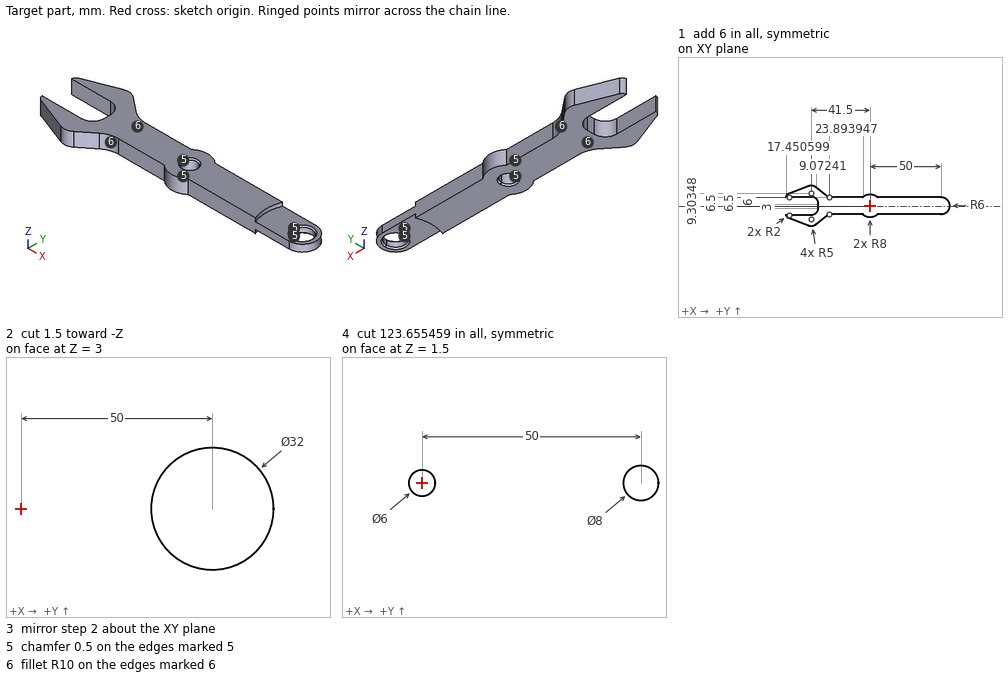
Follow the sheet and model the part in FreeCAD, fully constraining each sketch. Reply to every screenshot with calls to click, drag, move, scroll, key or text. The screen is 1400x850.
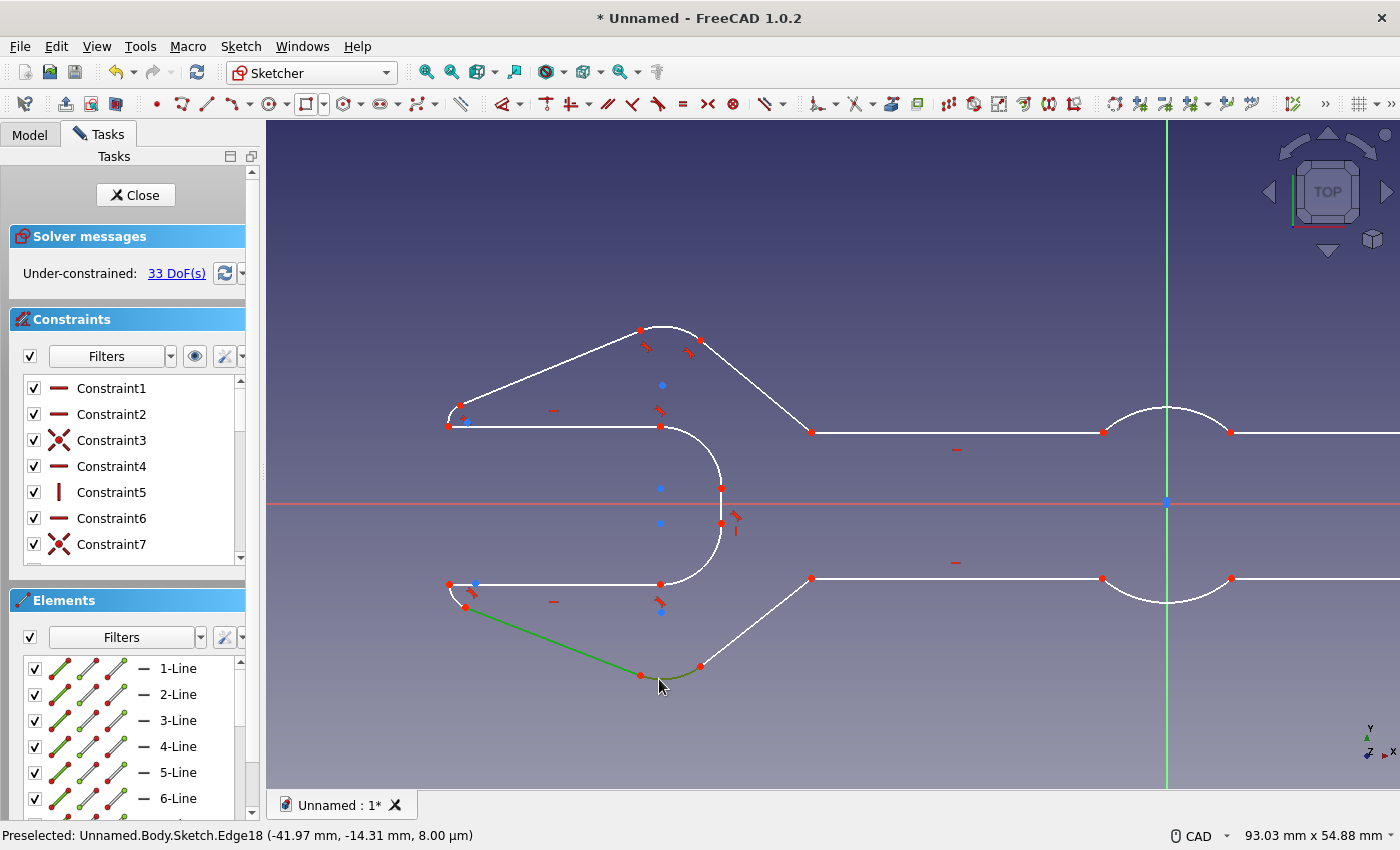
click(658, 104)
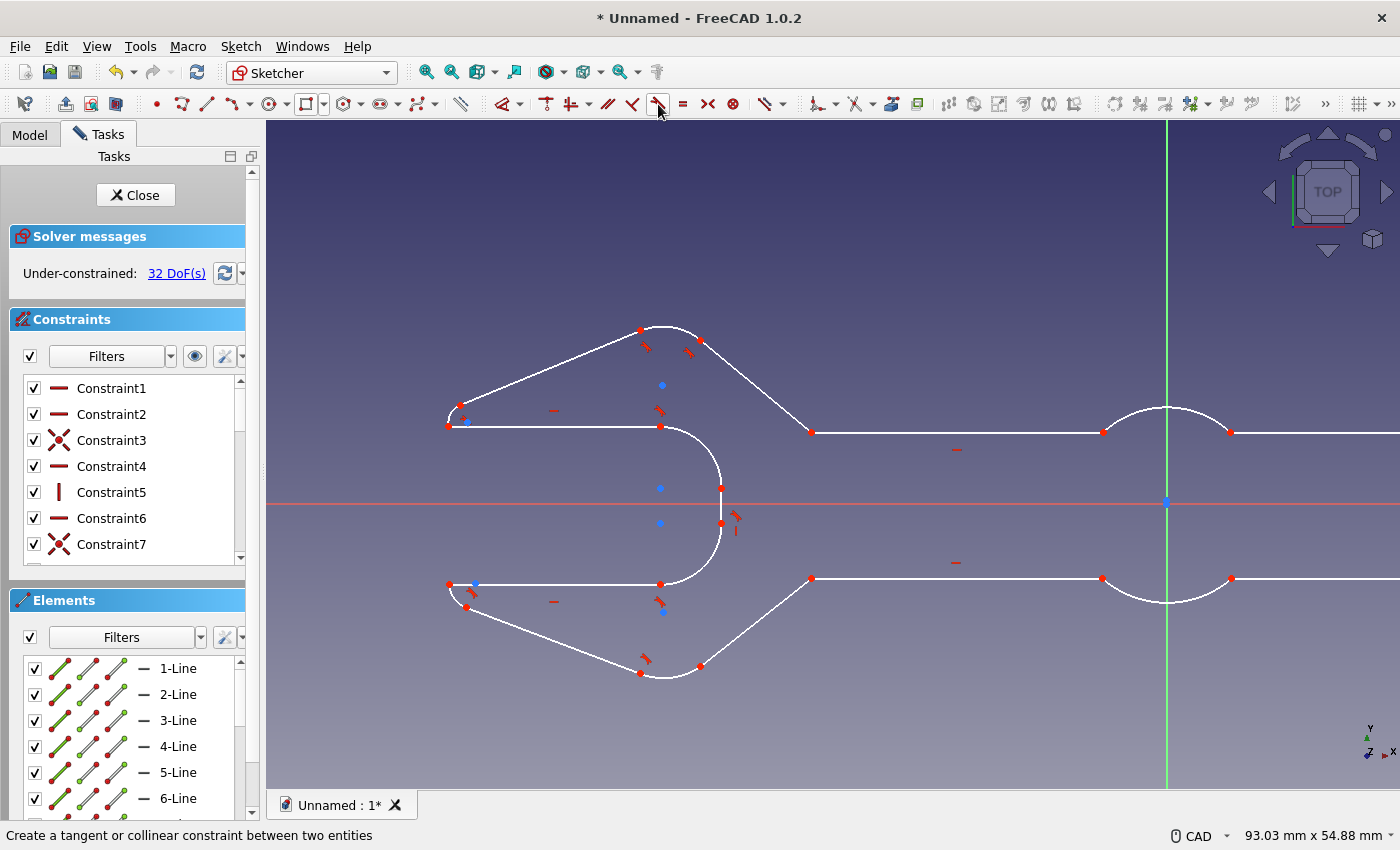
click(734, 640)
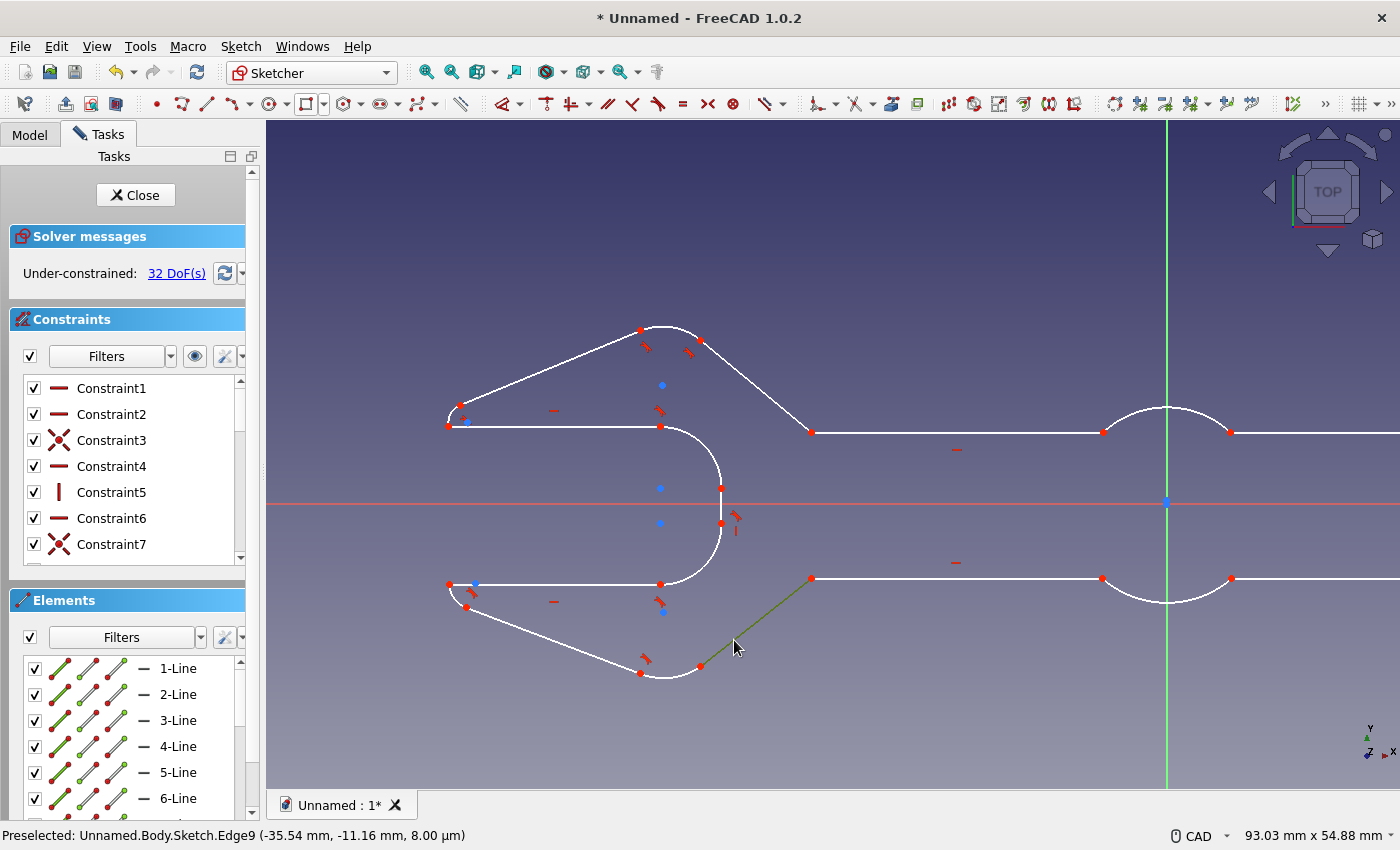
click(659, 678)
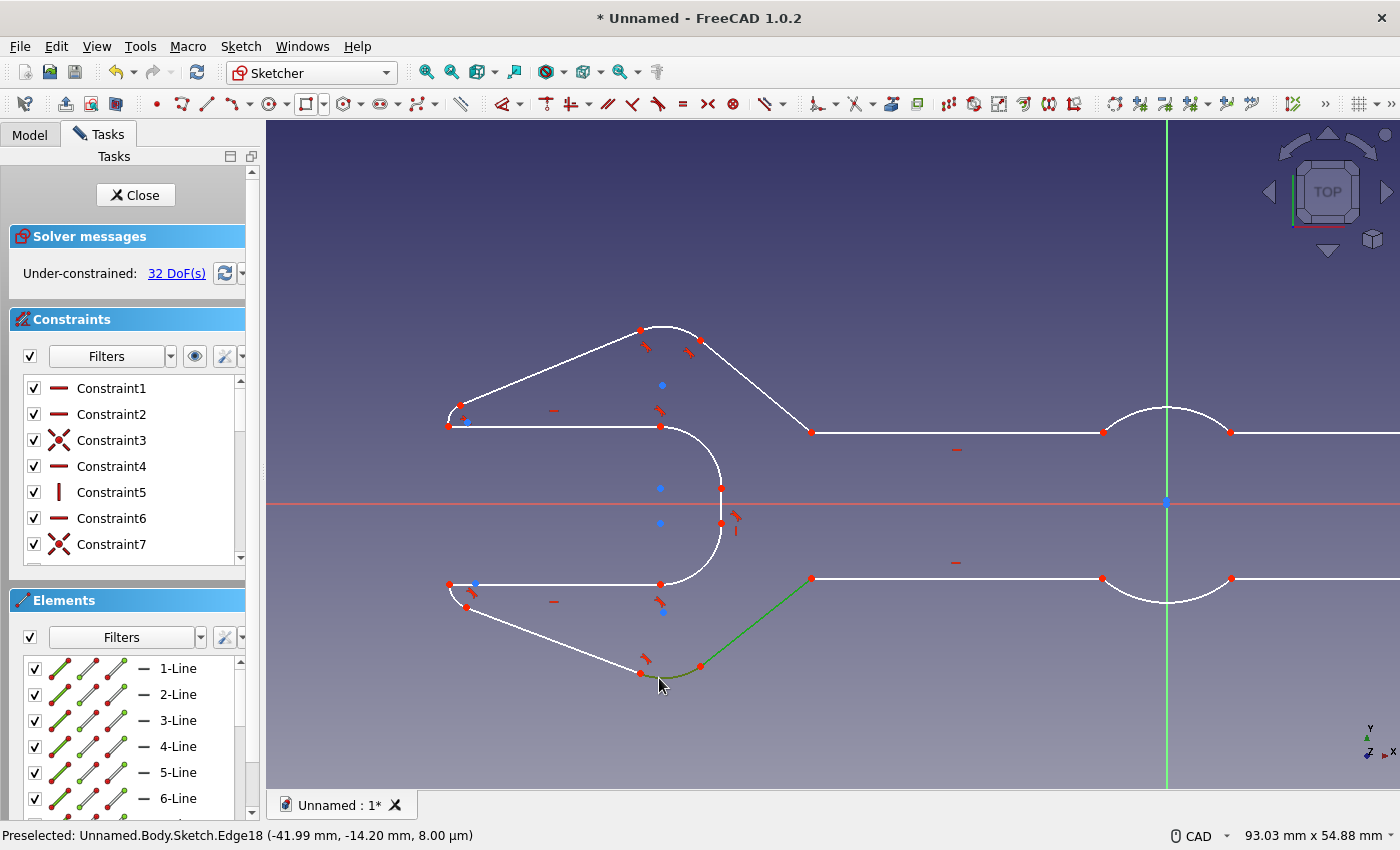
click(658, 104)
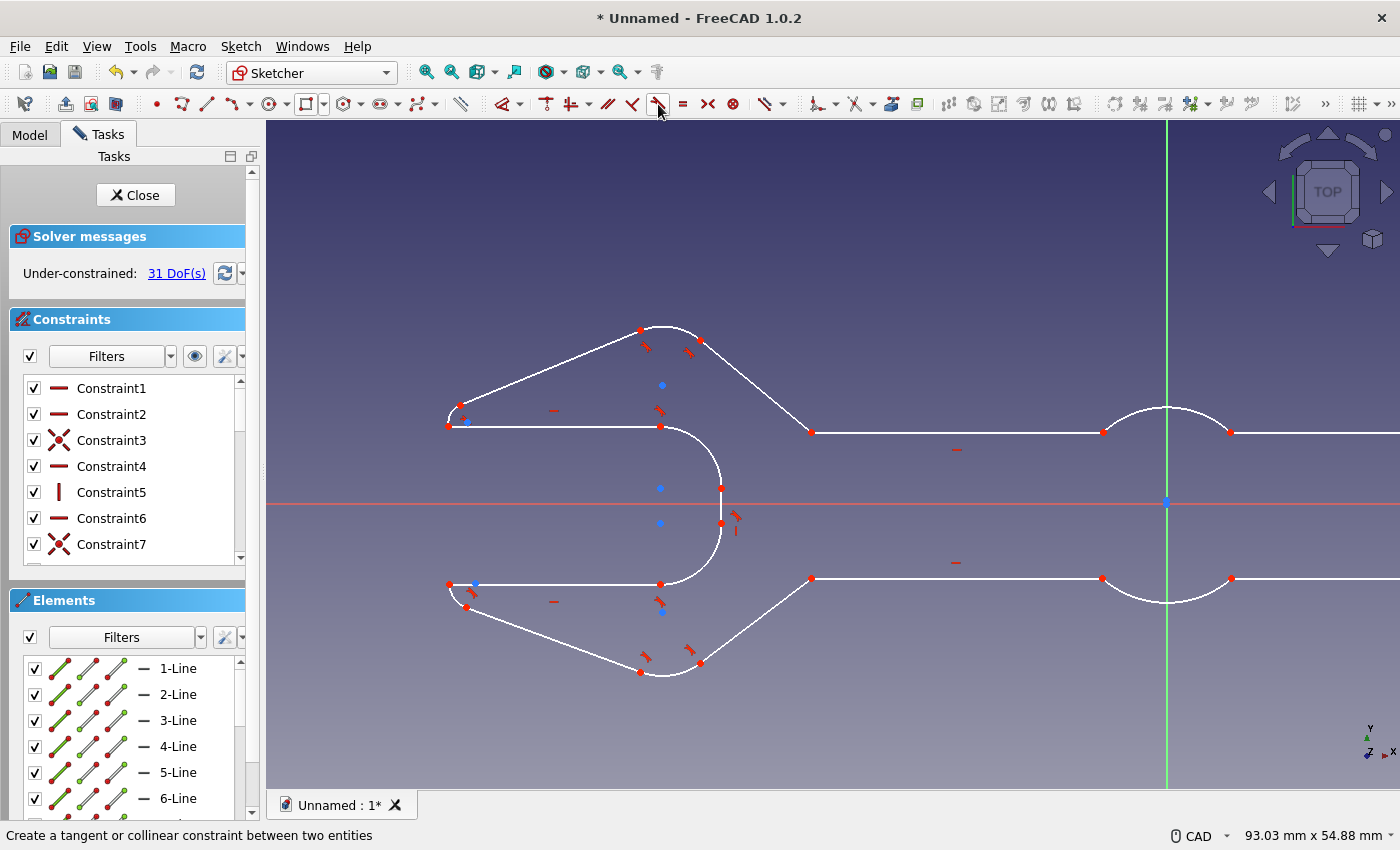
scroll(451, 414, down, 4)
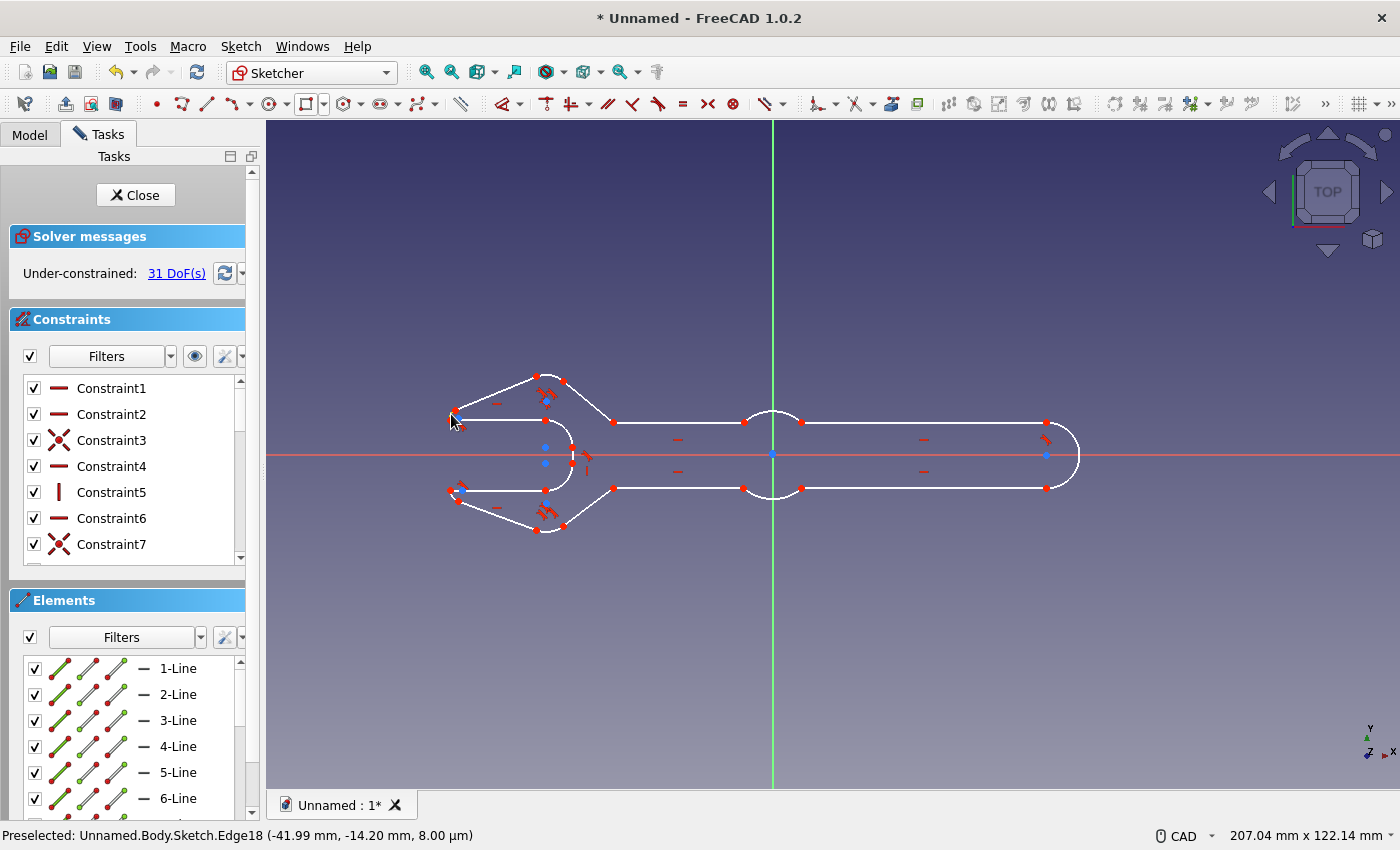
click(875, 488)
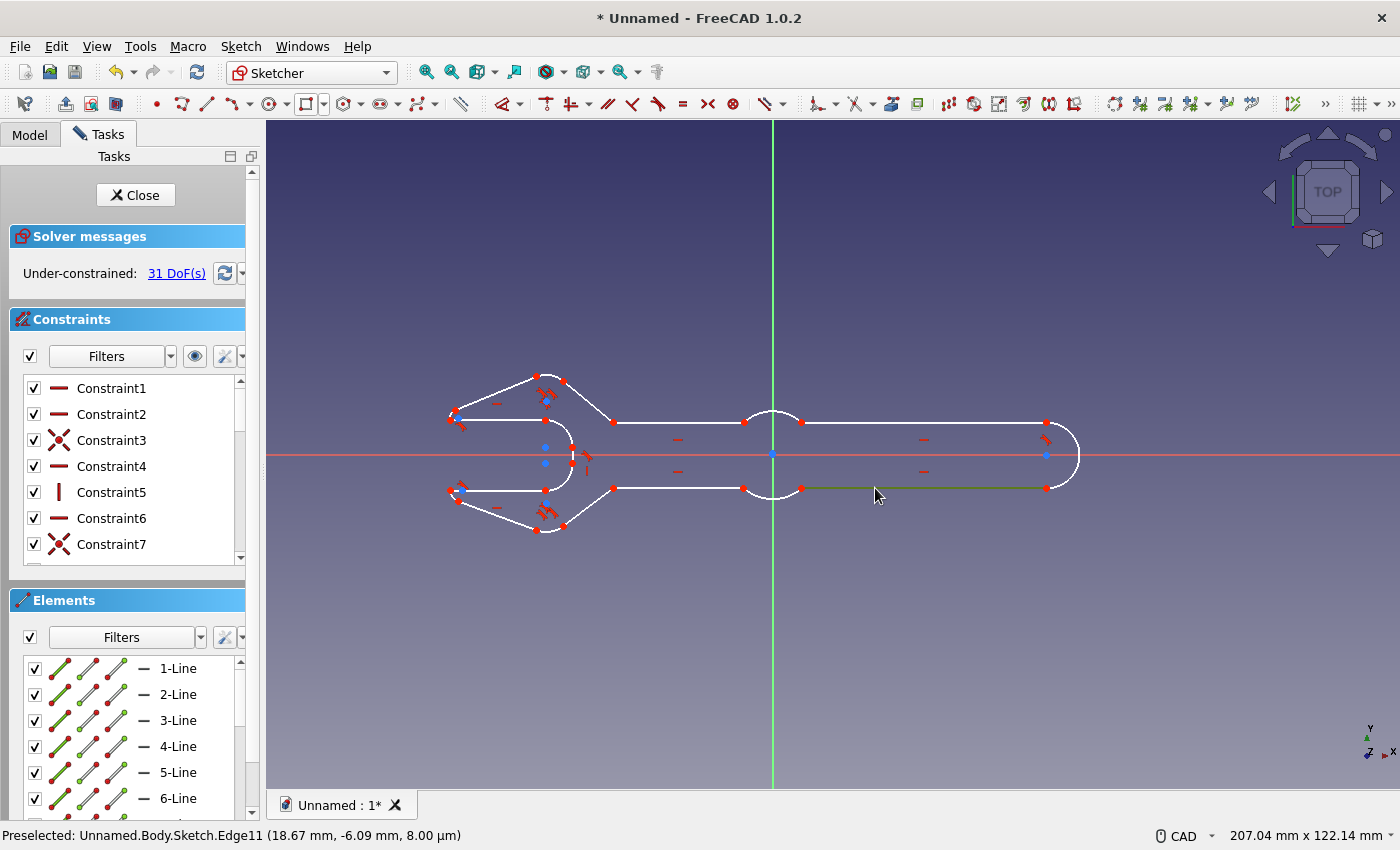
click(1073, 475)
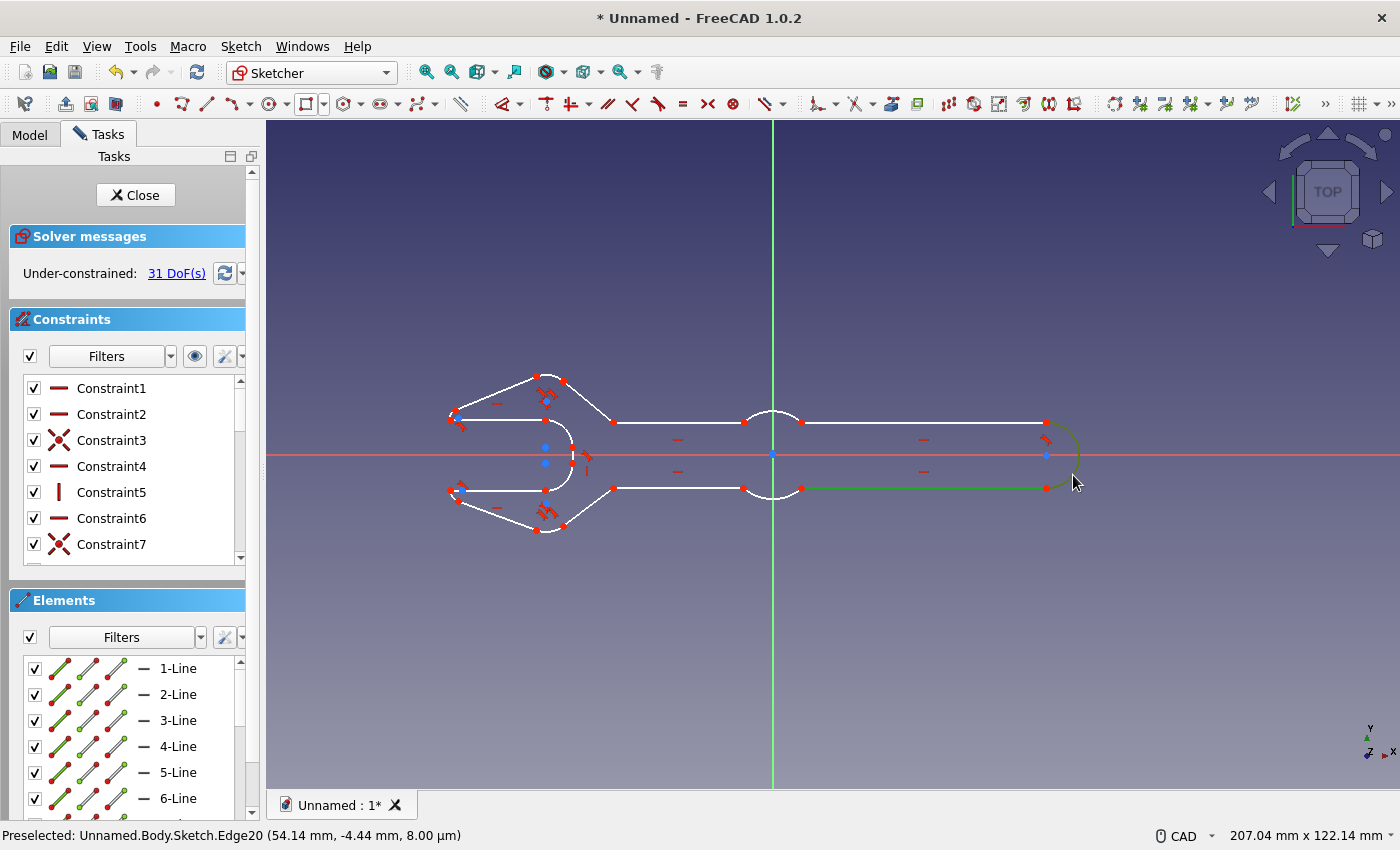
click(658, 104)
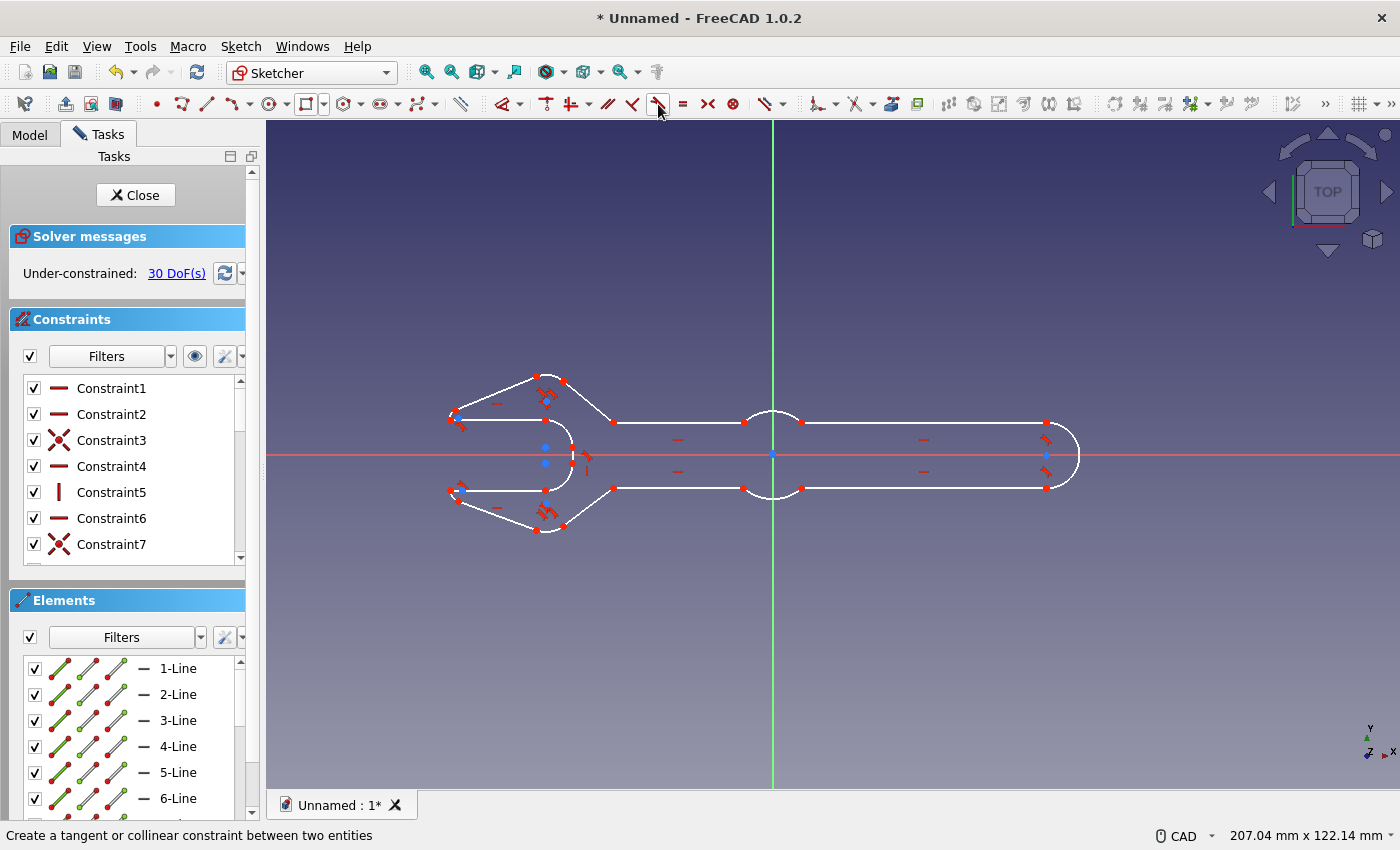
click(785, 413)